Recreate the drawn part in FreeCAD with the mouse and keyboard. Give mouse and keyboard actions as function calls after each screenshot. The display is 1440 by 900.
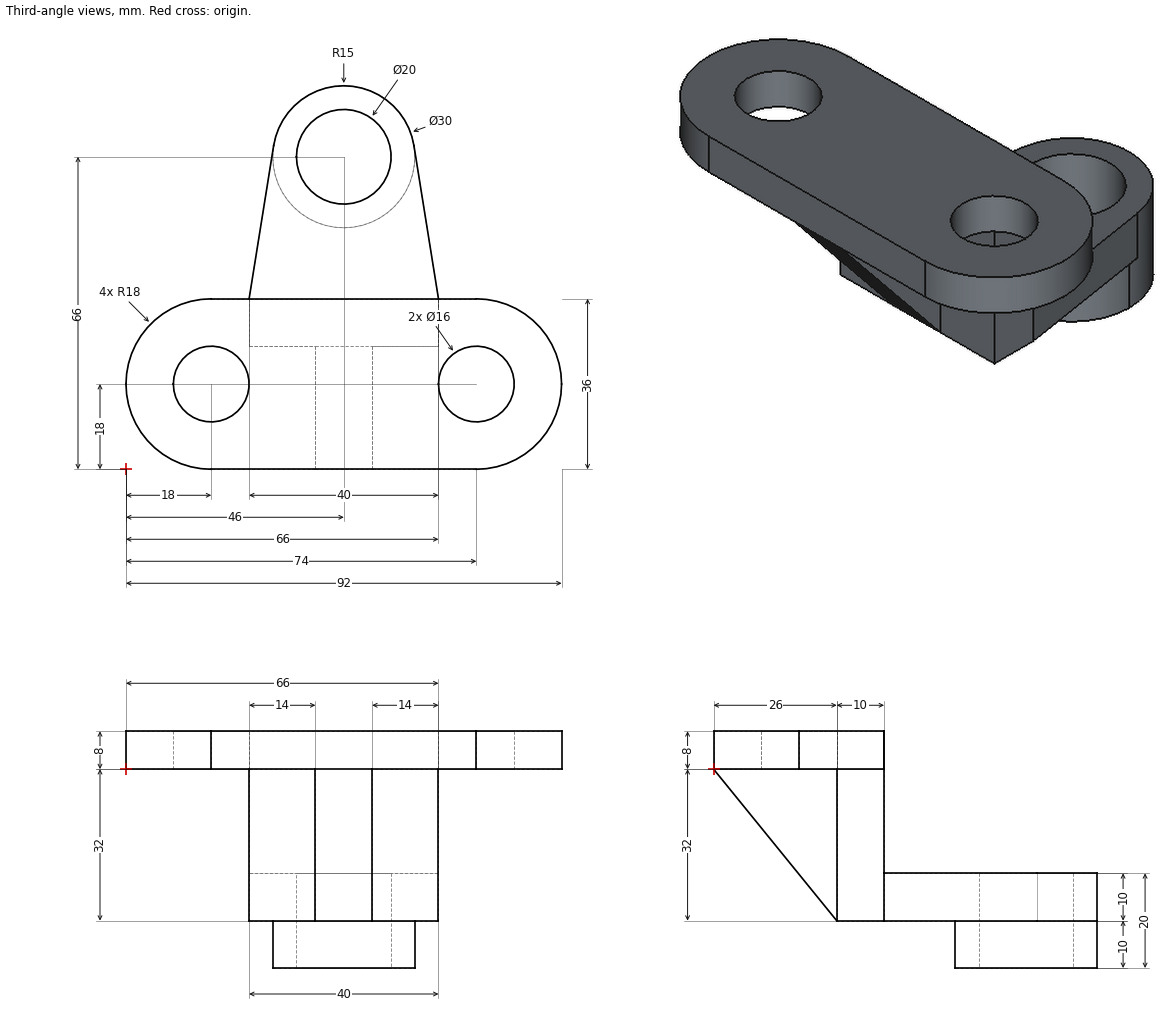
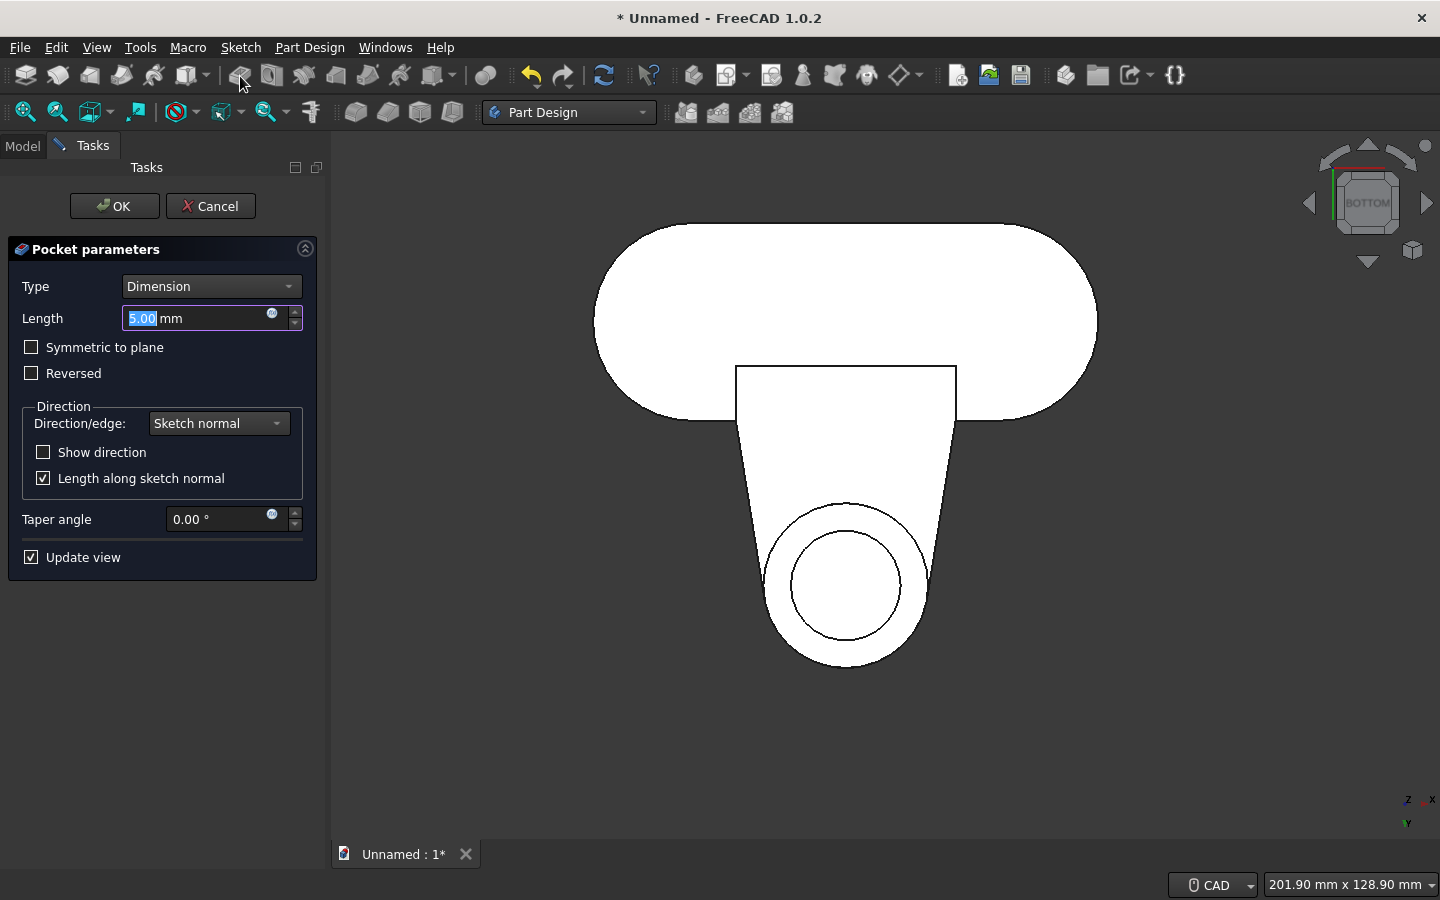
text(20)
key(Tab)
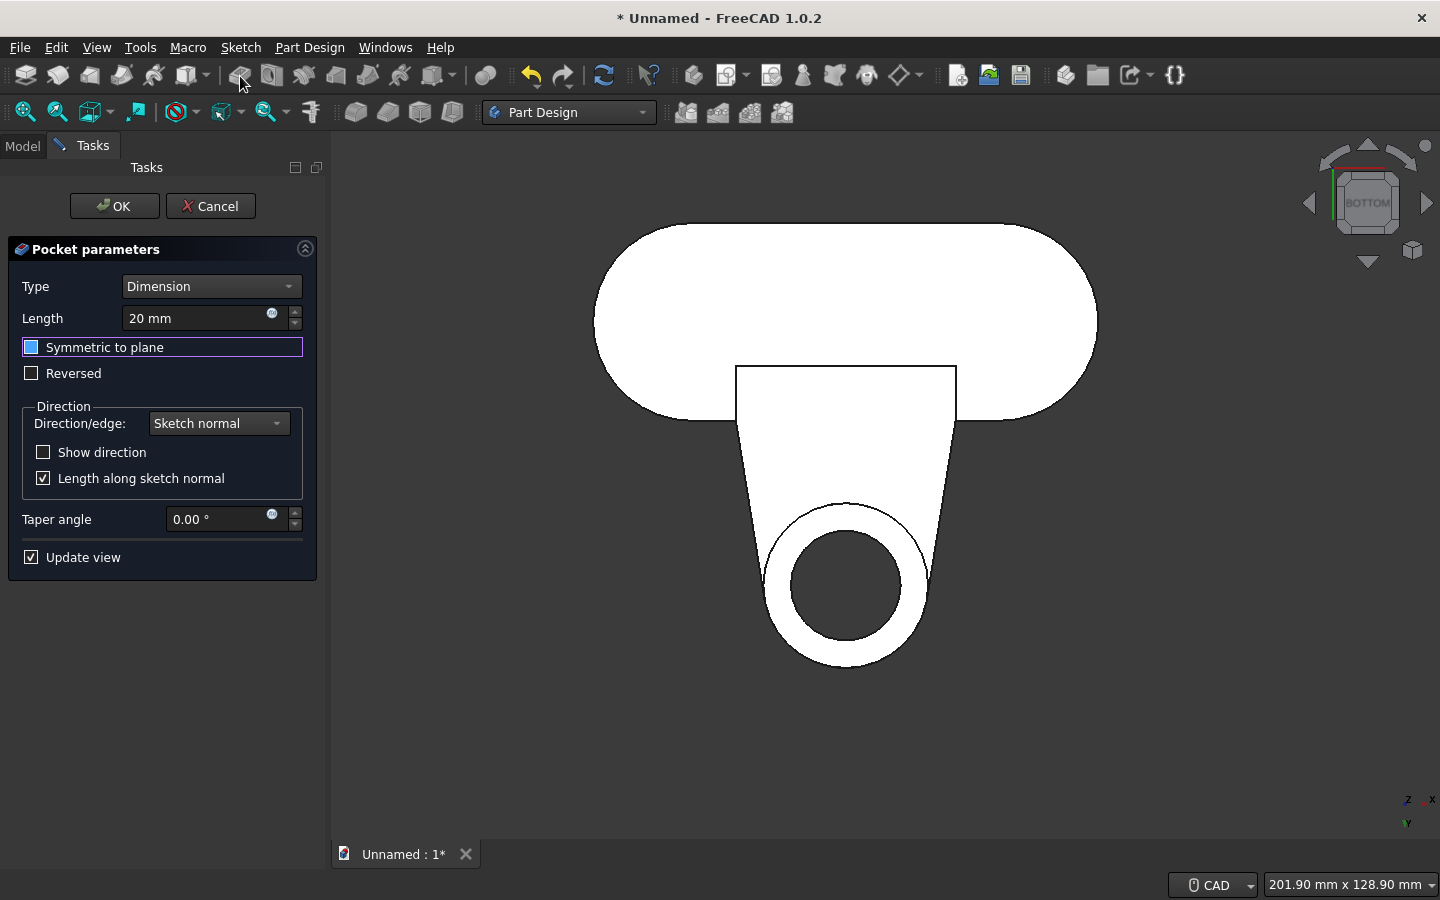
click(115, 206)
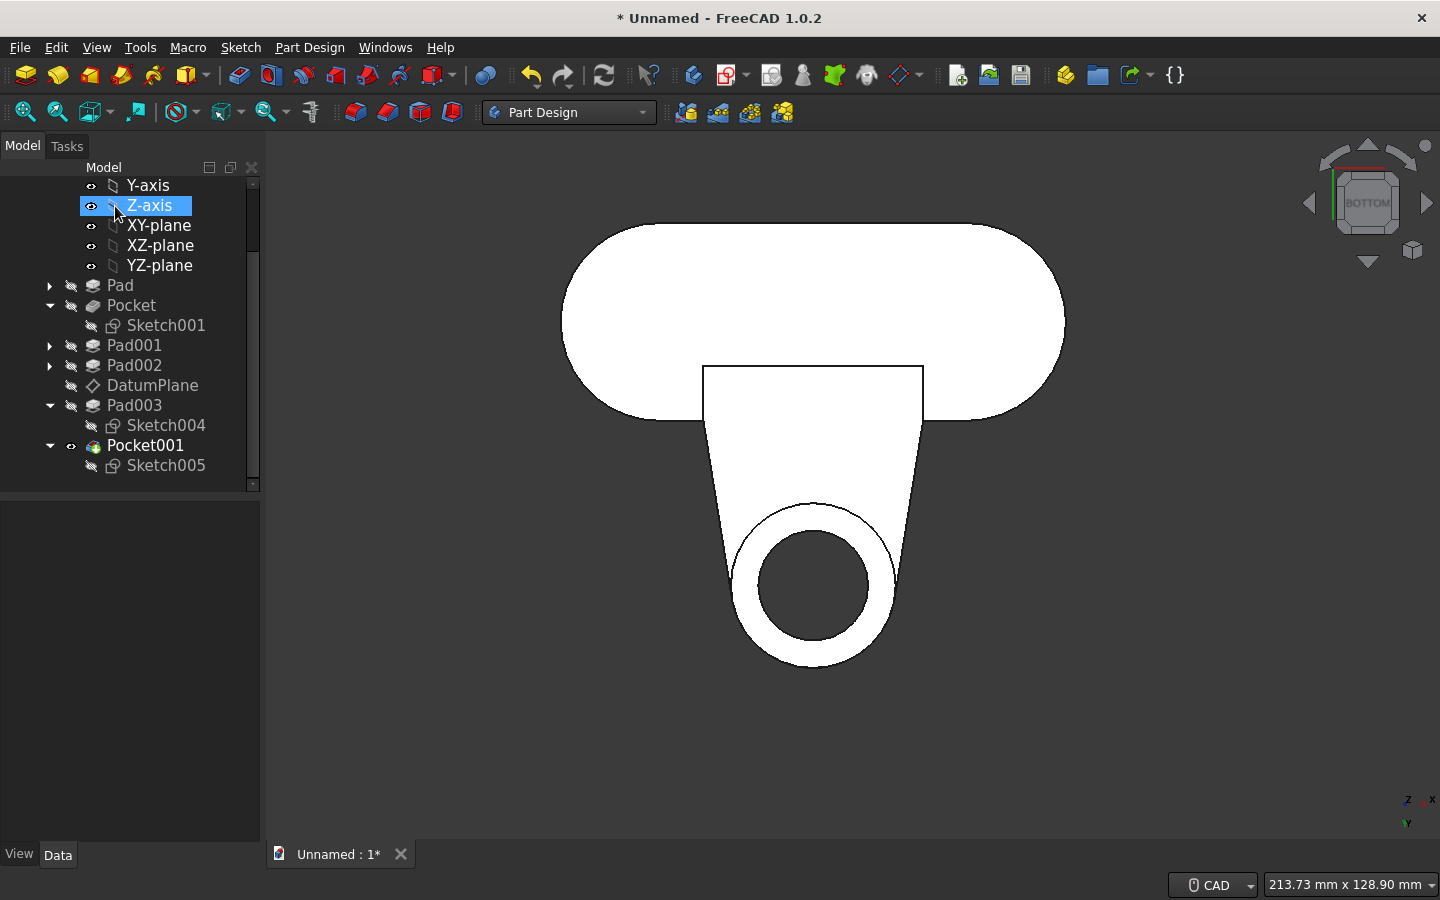
click(958, 293)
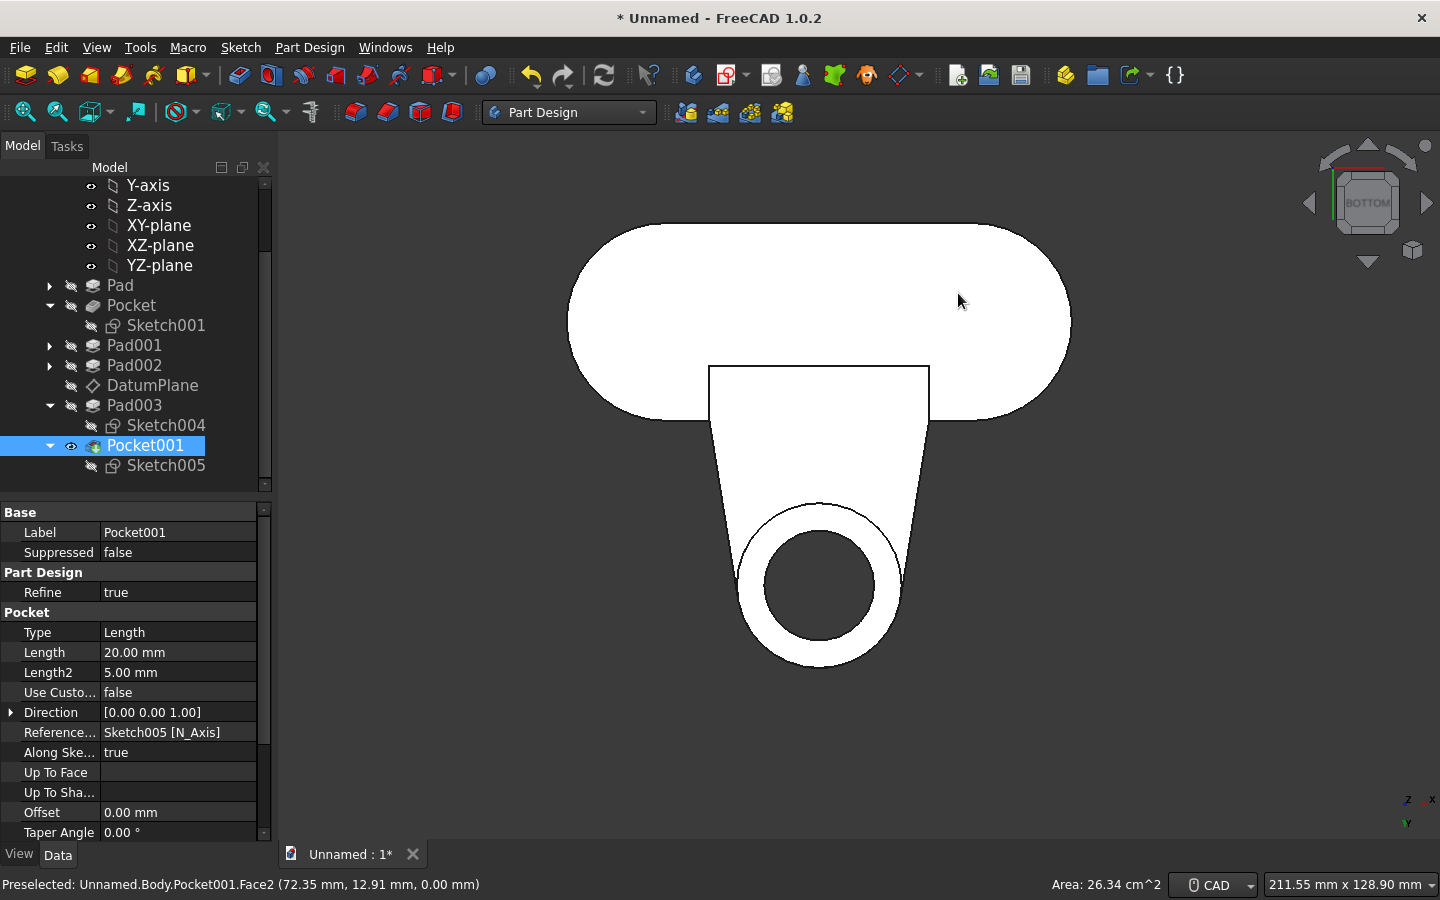
click(726, 76)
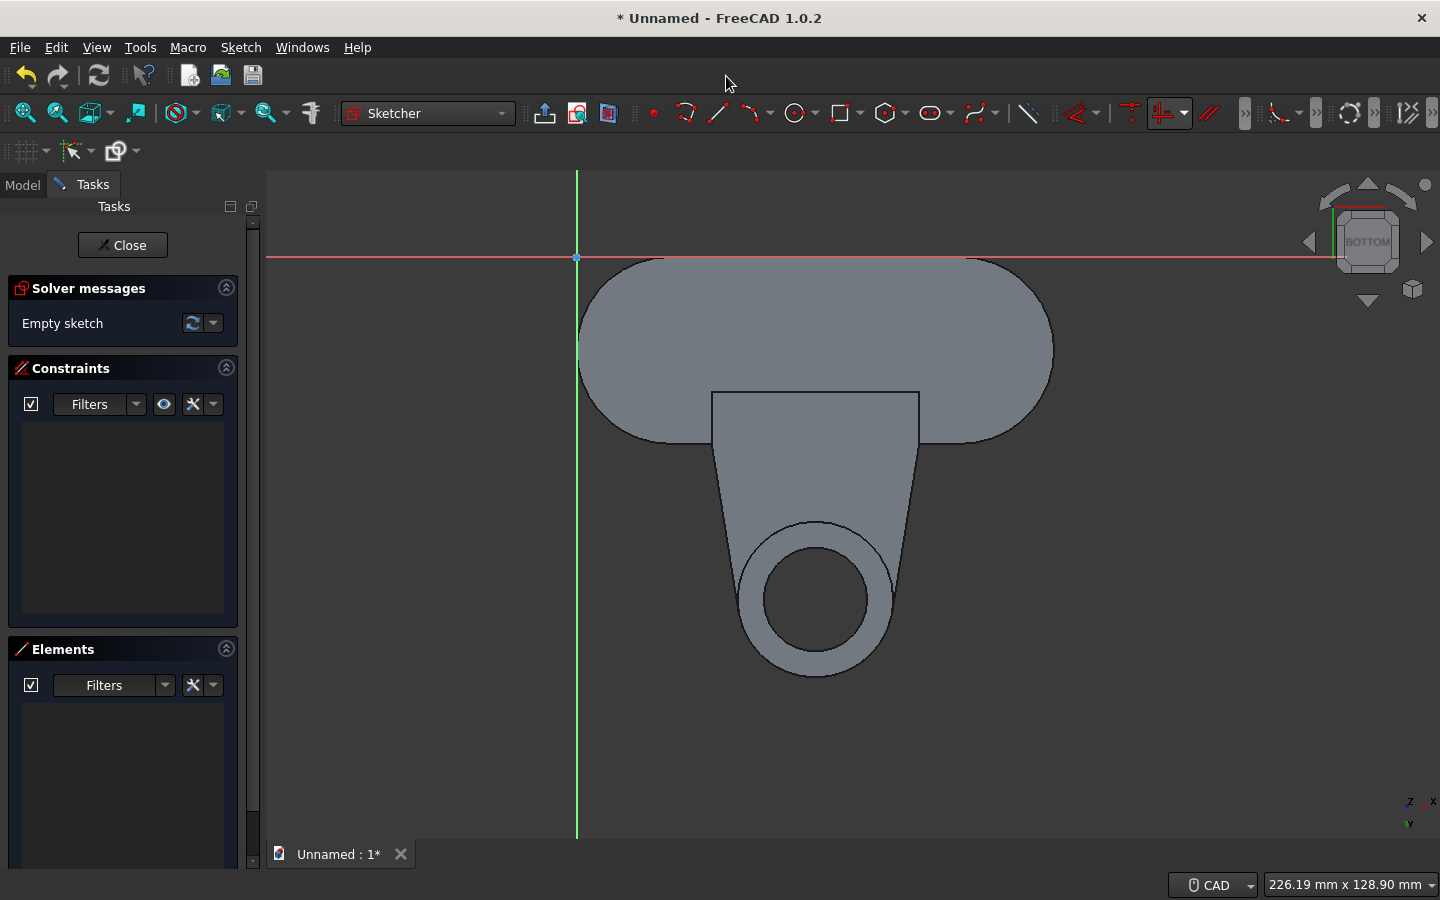
scroll(800, 198, up, 2)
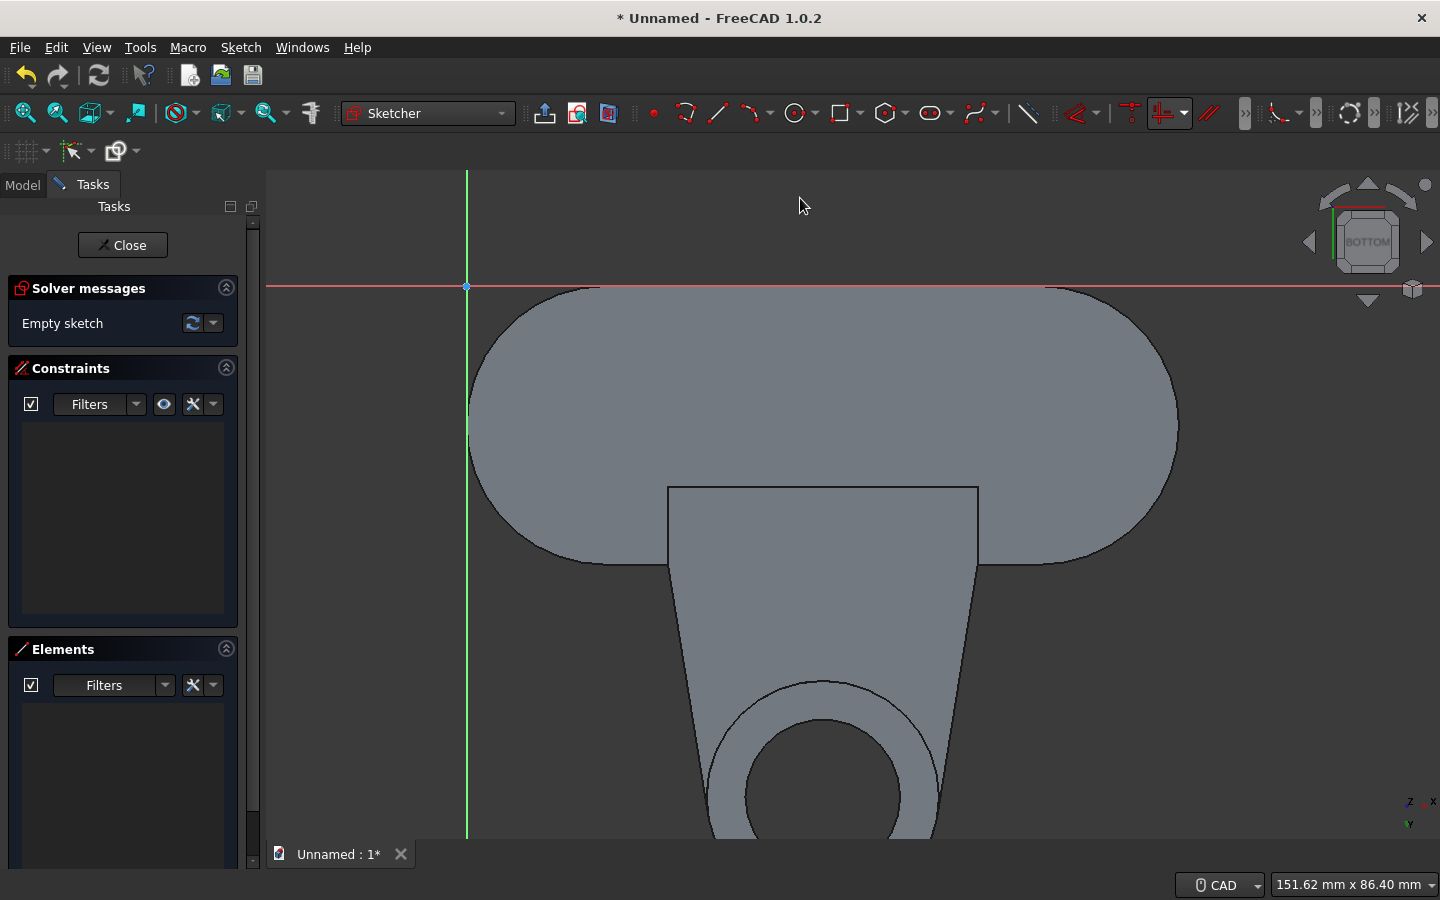
click(796, 114)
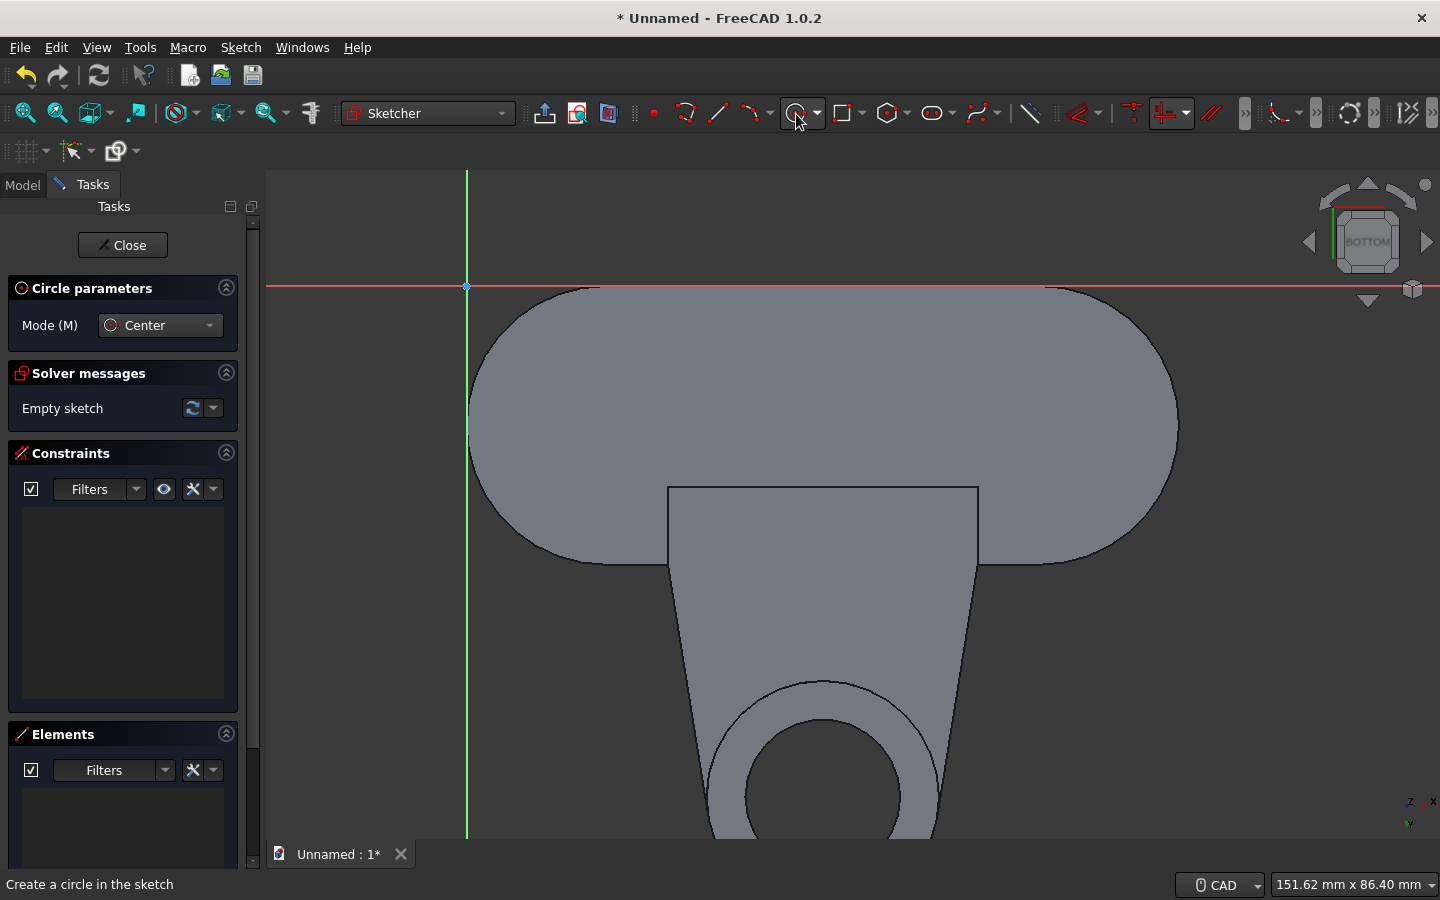
click(1040, 425)
move(1083, 382)